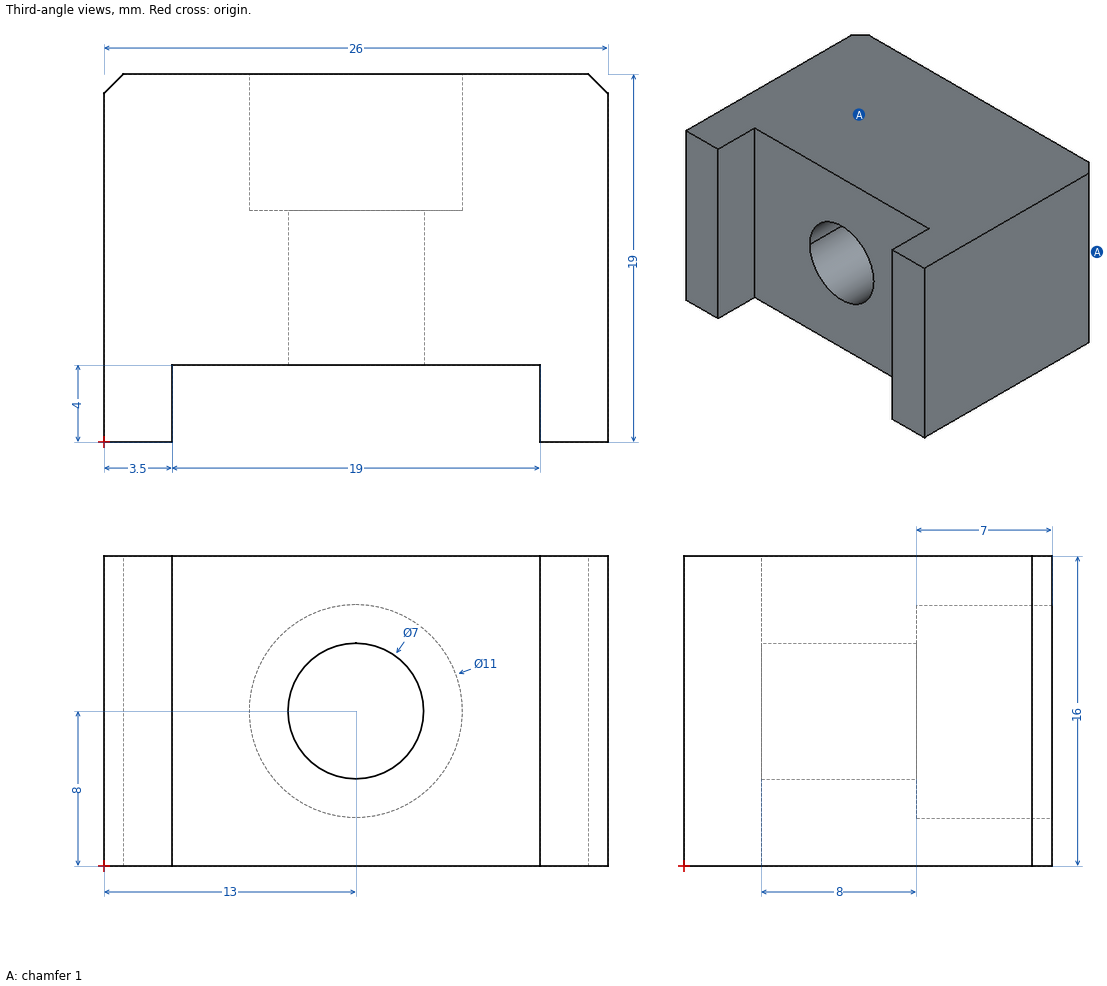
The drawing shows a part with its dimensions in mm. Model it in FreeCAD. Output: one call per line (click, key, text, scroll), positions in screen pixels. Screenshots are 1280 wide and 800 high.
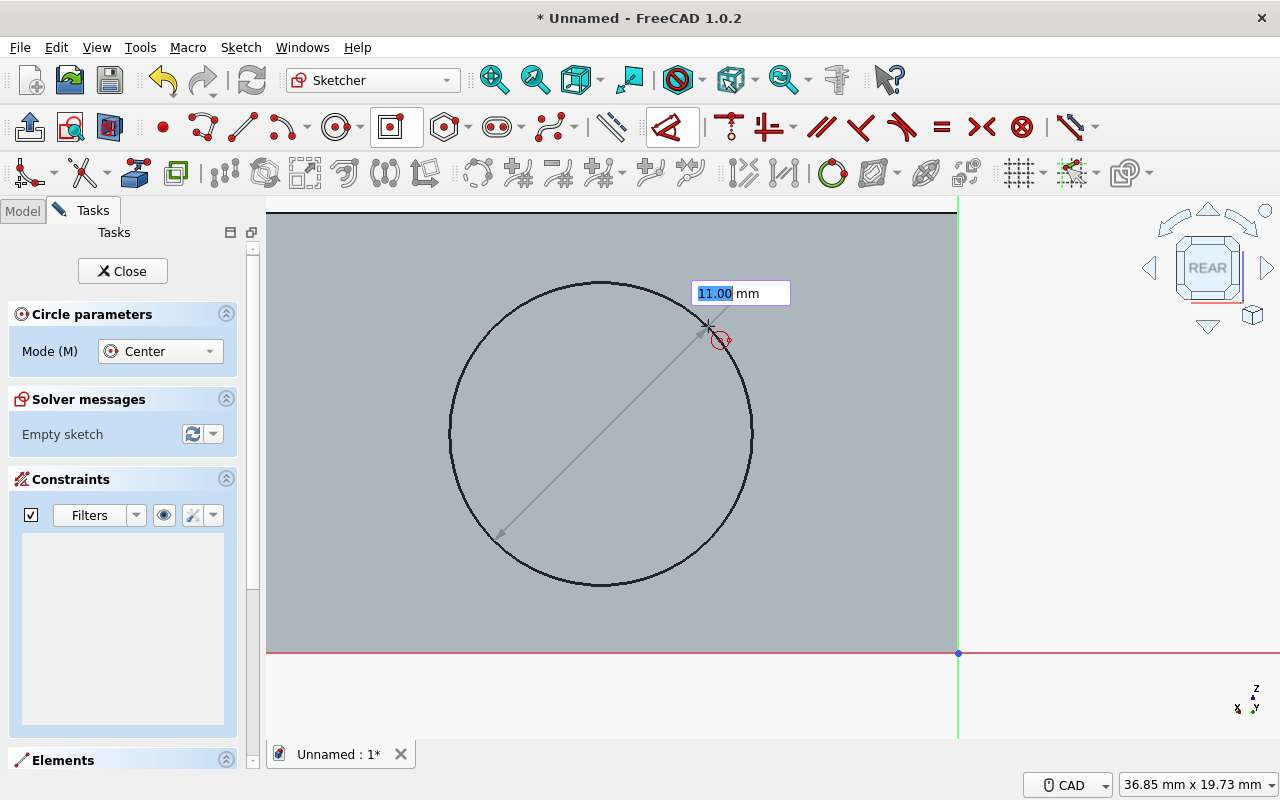
text(11)
key(Return)
key(Escape)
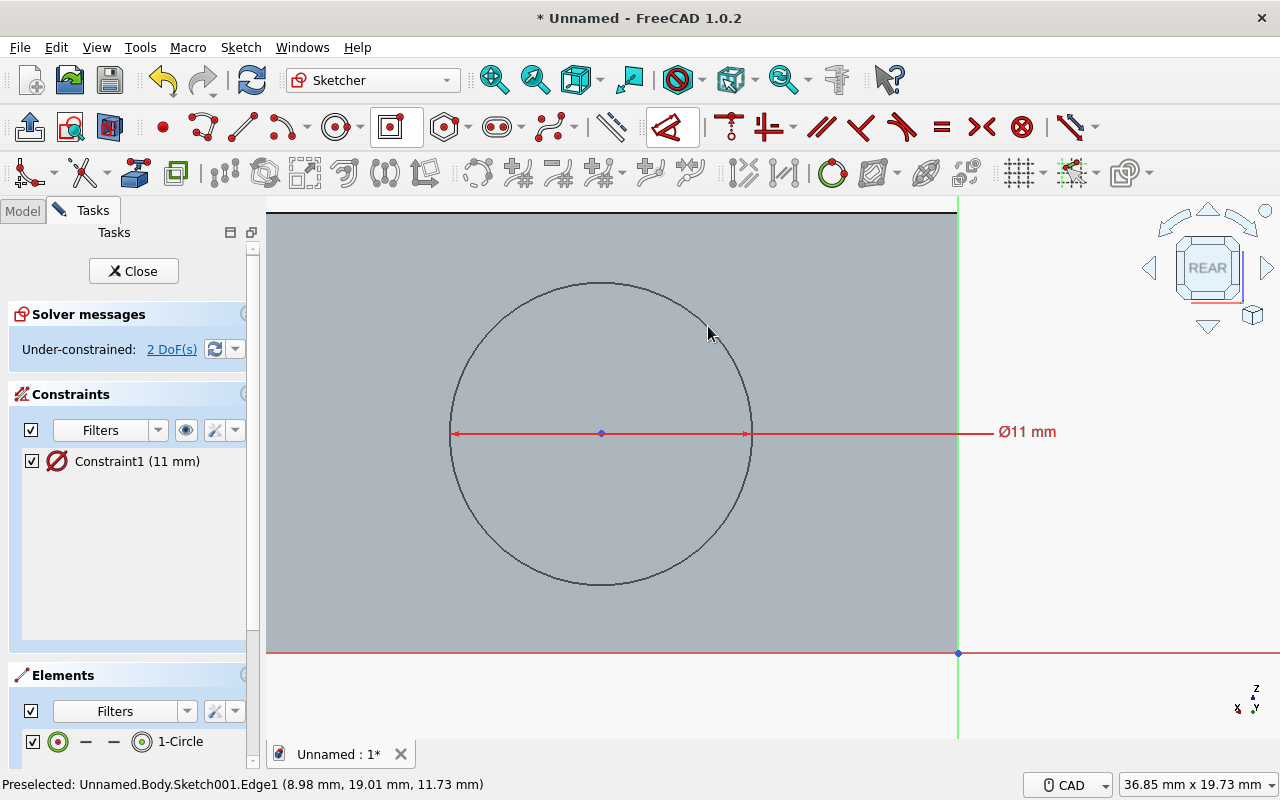
click(601, 434)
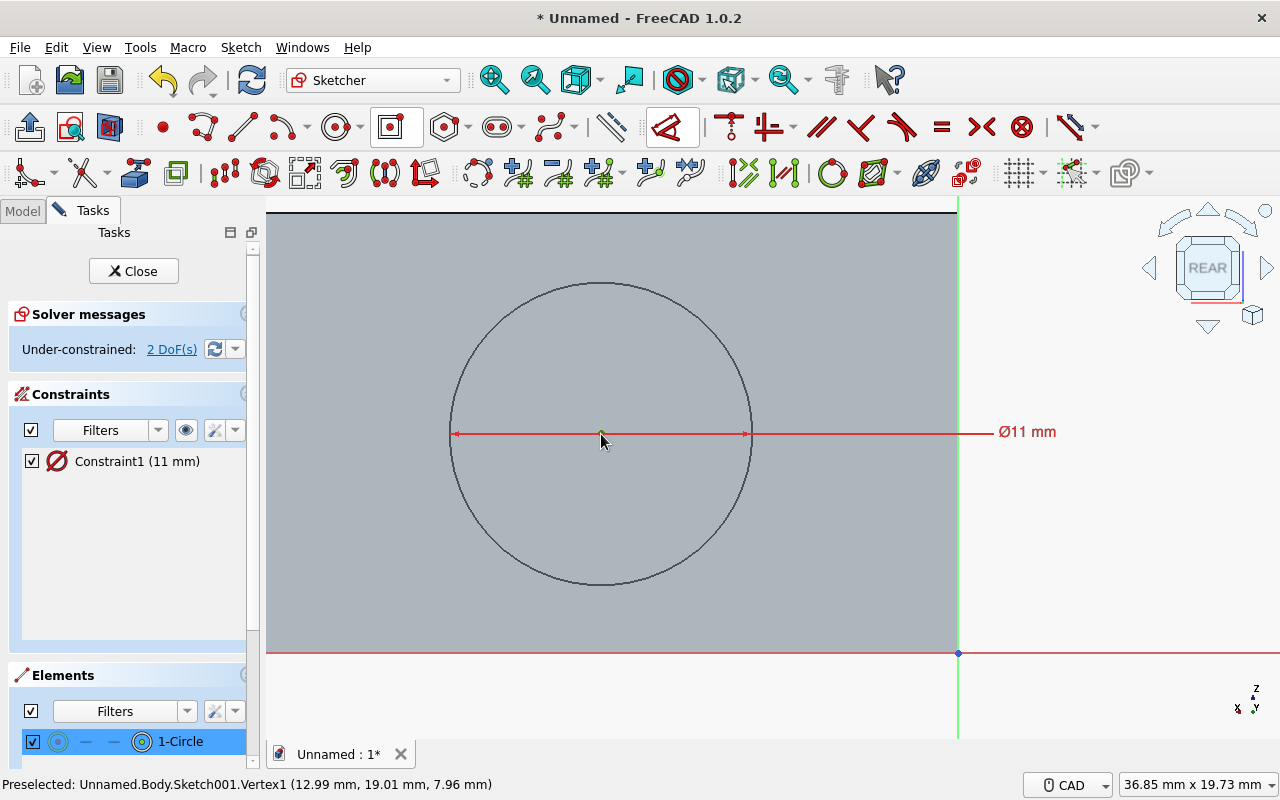
click(694, 128)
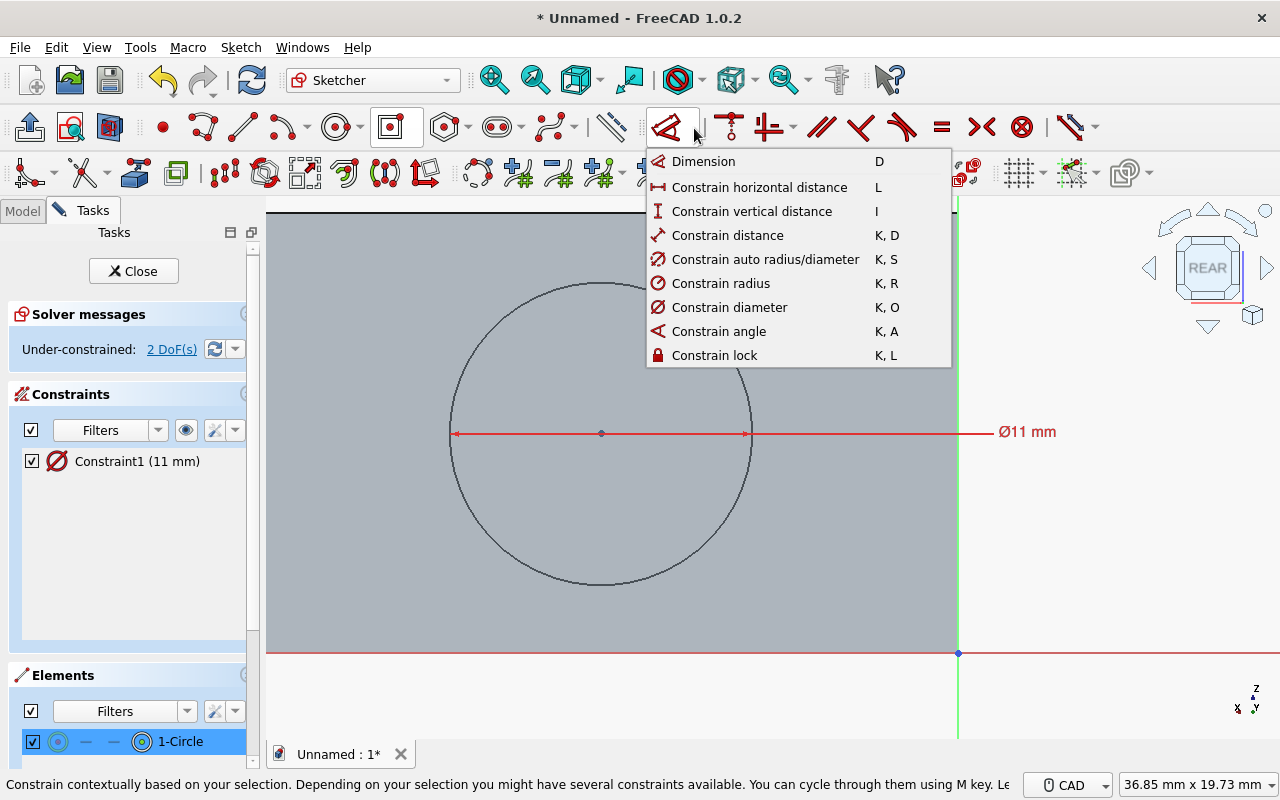
click(799, 211)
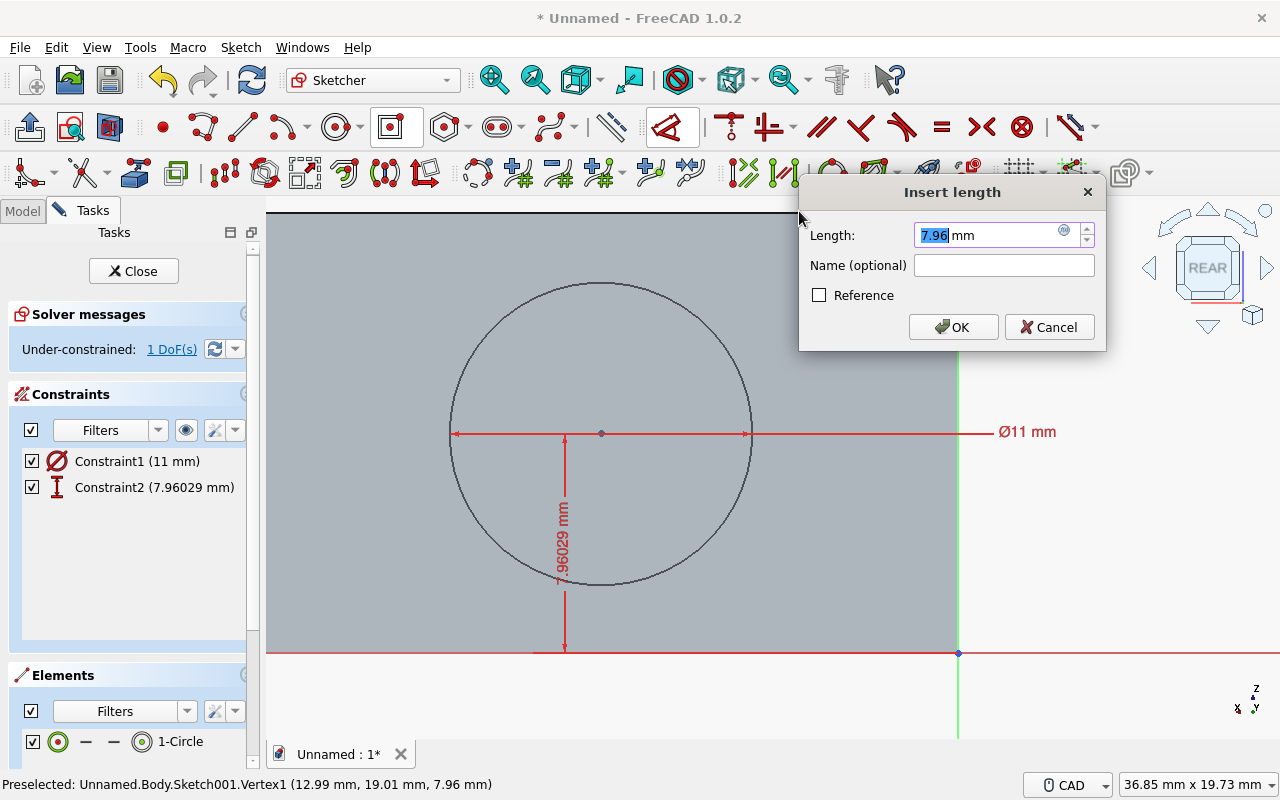
text(8)
key(Return)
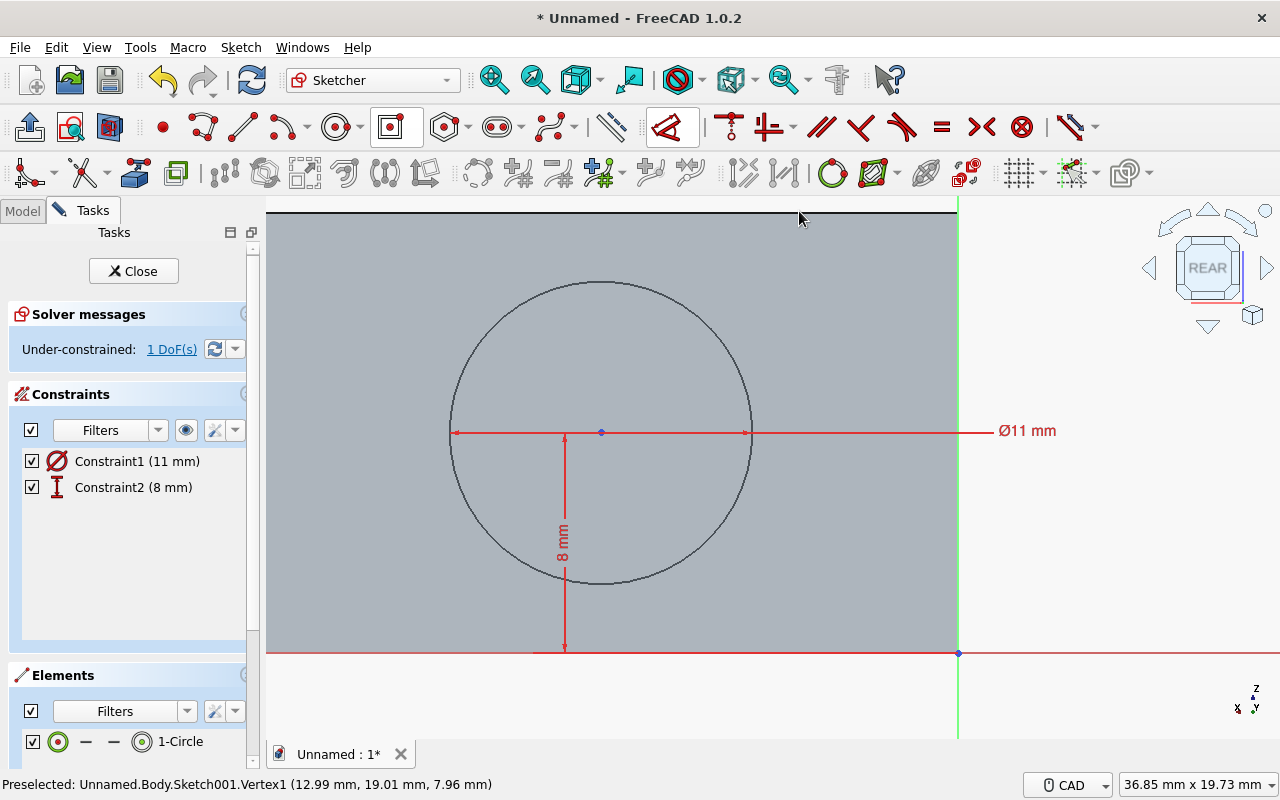
click(601, 433)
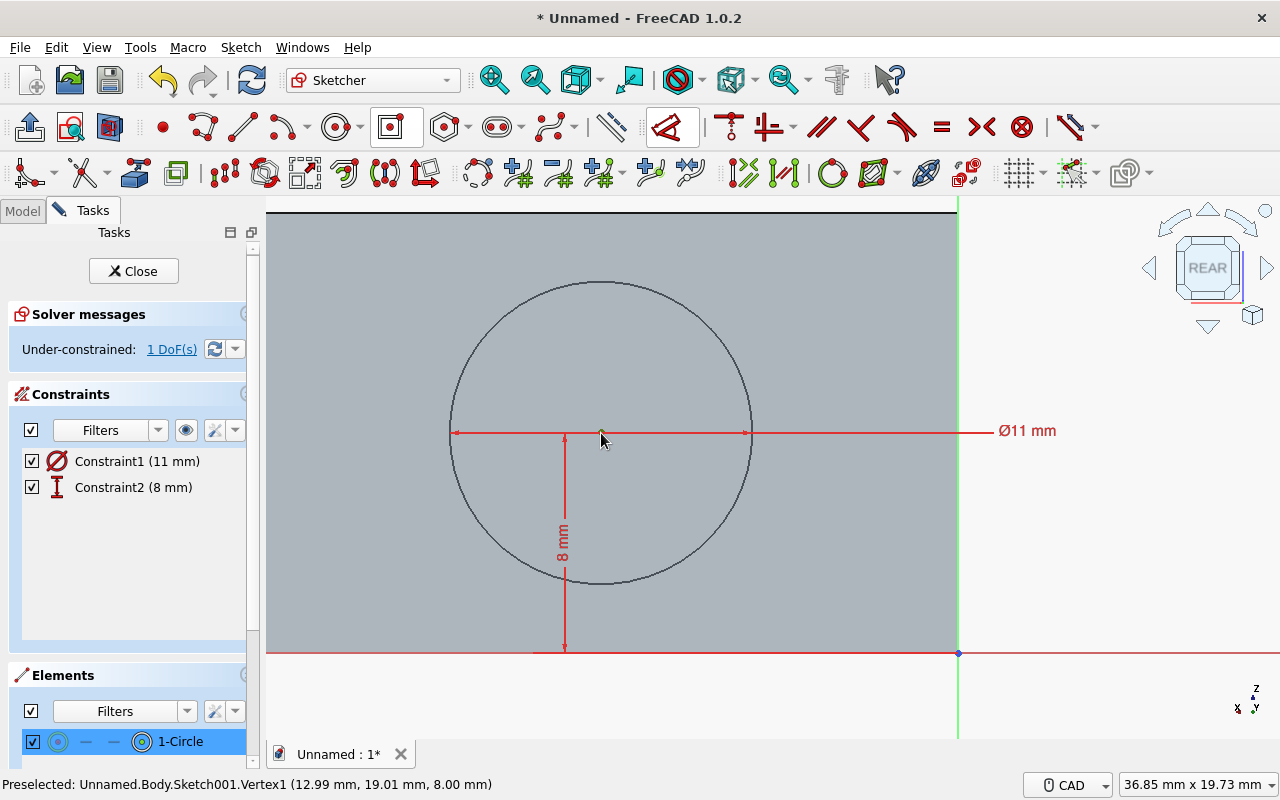
key(l)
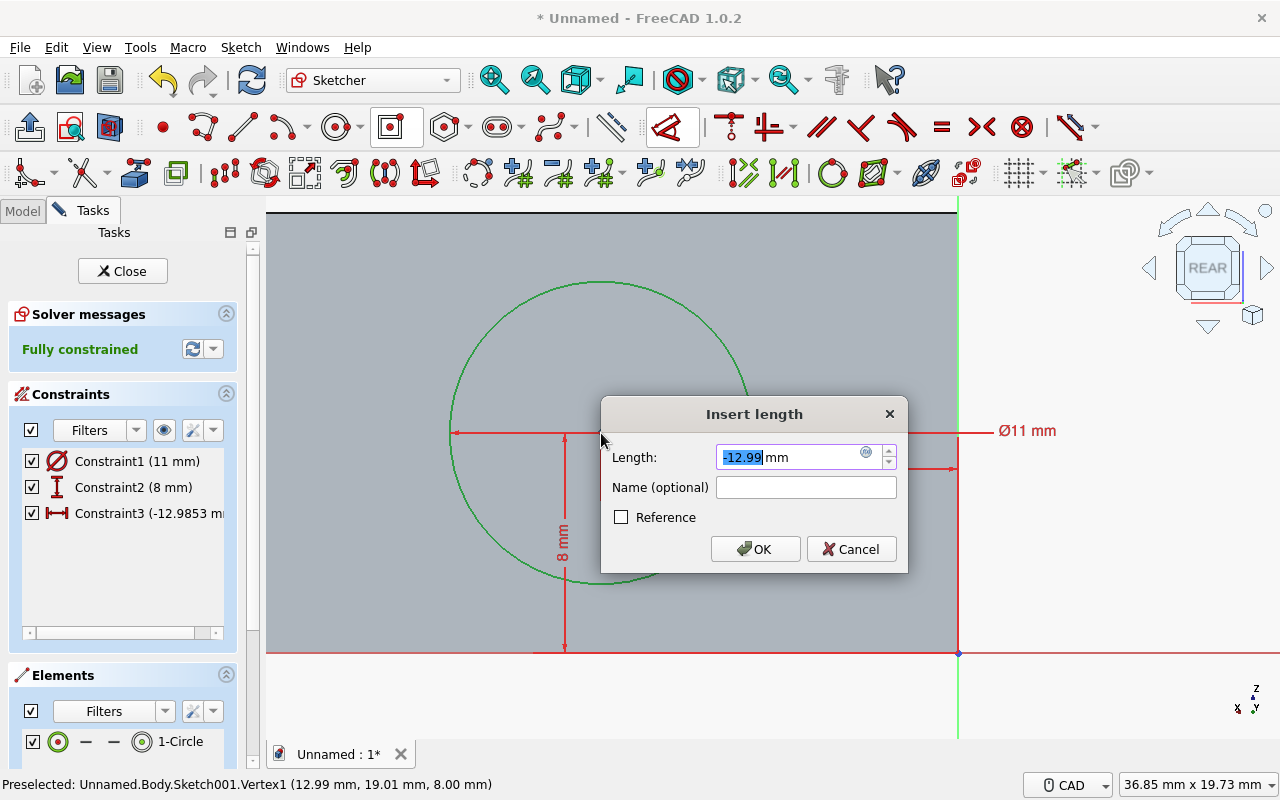
text(-13)
key(Return)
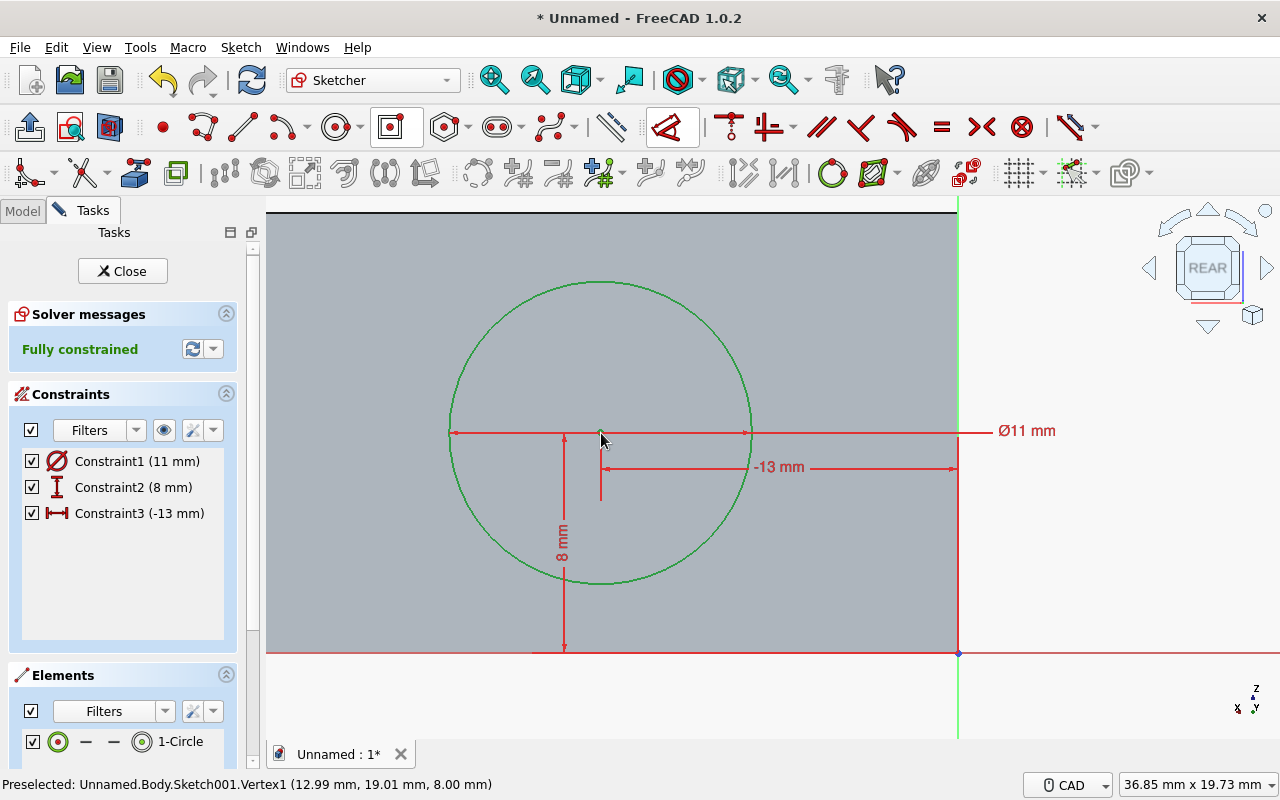
click(123, 271)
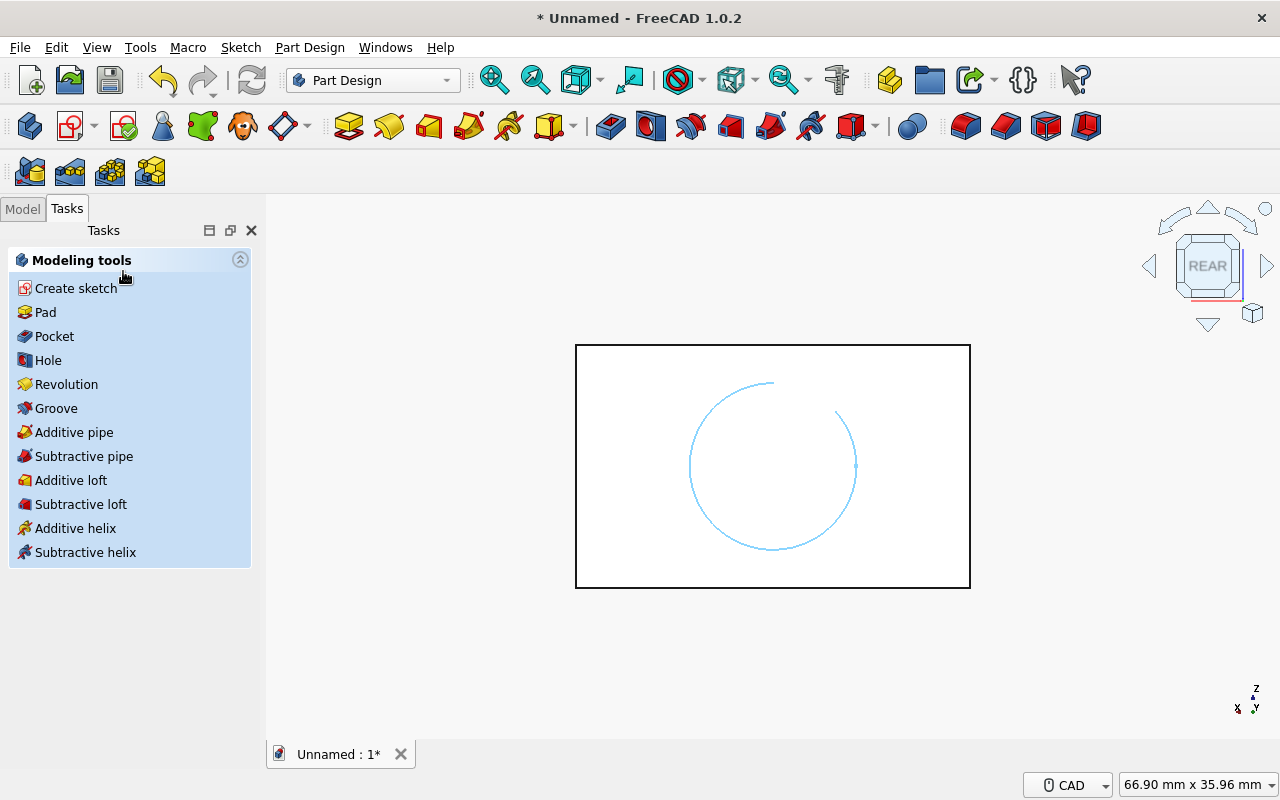
click(612, 126)